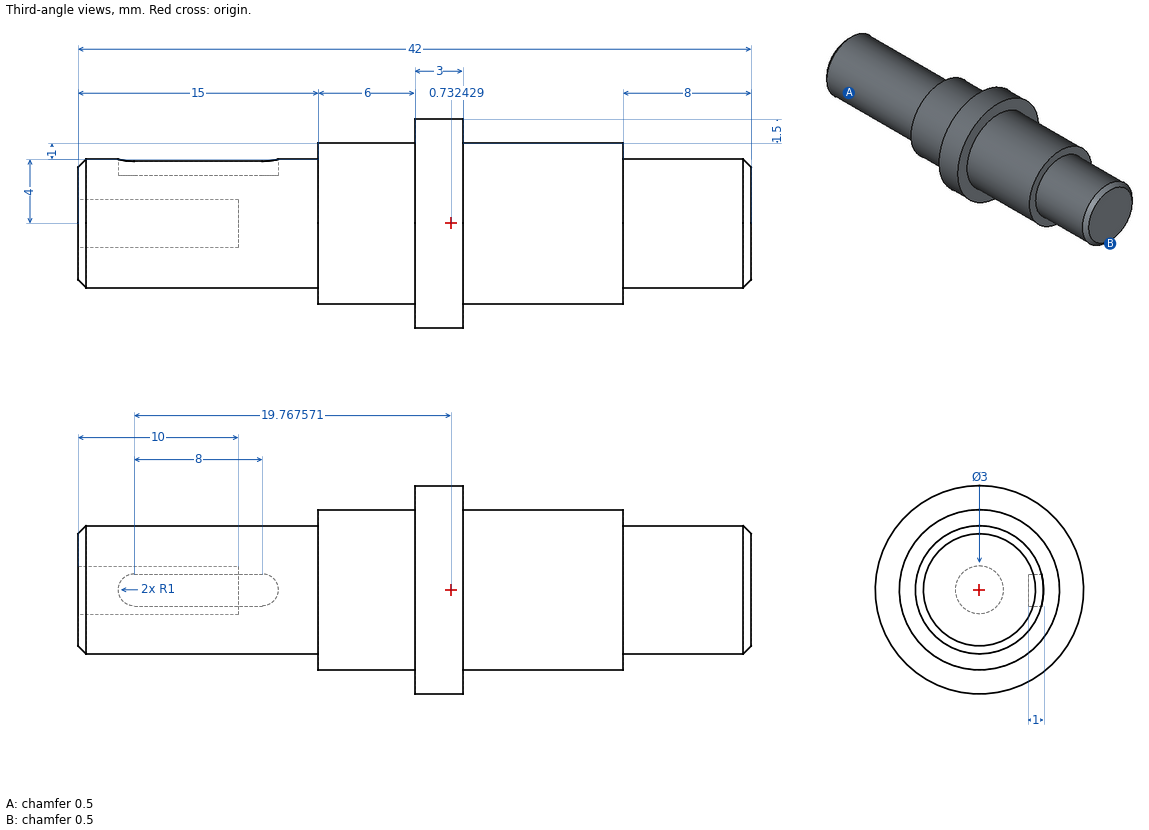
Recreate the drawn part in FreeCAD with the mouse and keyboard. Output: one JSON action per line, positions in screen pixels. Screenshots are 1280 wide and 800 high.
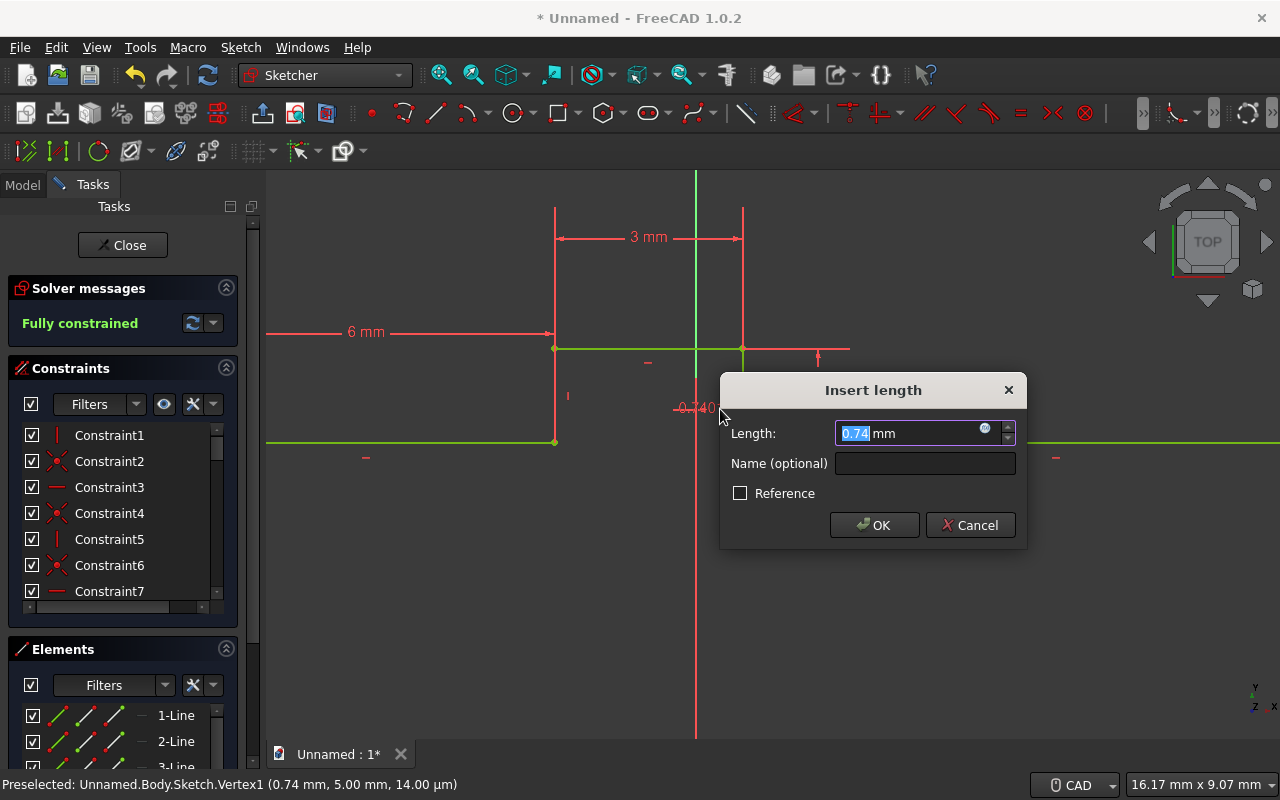
{"action": "type", "text": "0.732429"}
{"action": "key", "text": "Return"}
{"action": "key", "text": "Escape"}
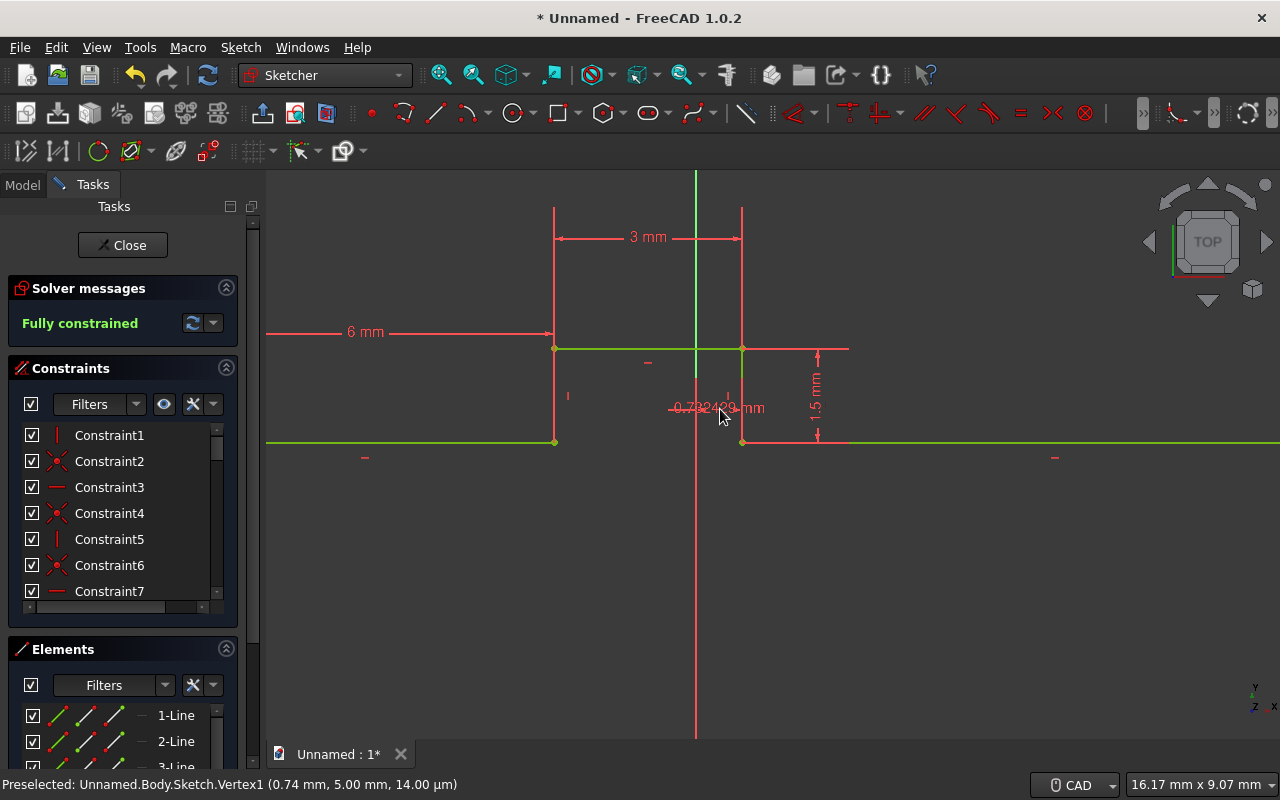
{"action": "left_click", "coordinate": [123, 245]}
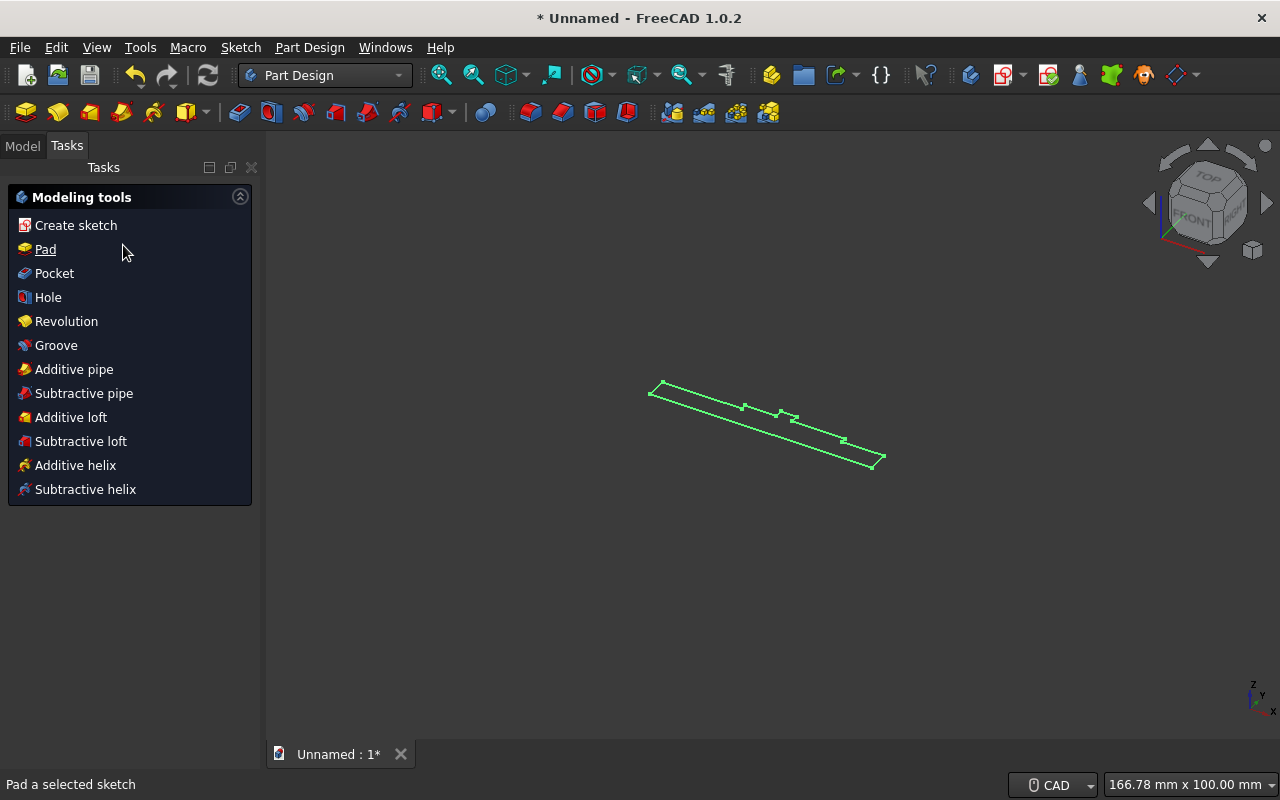
{"action": "left_click", "coordinate": [58, 112]}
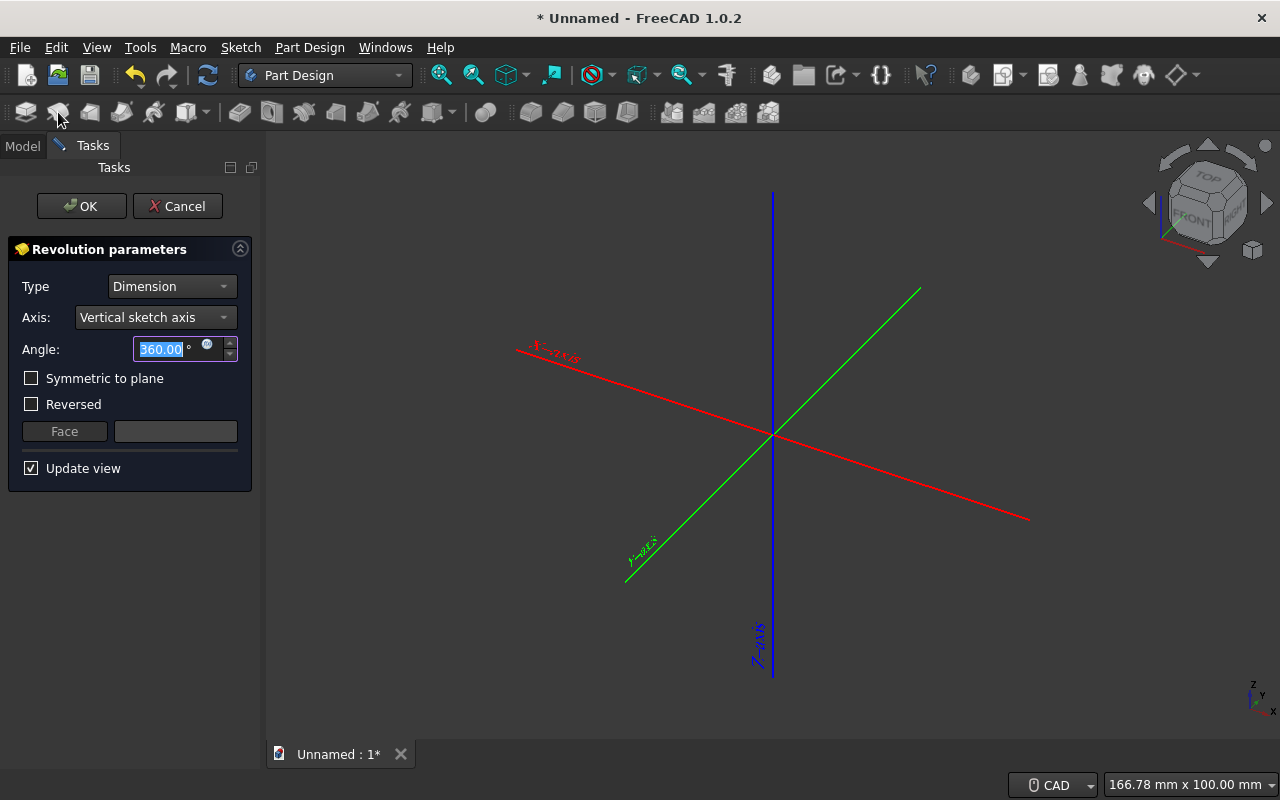
{"action": "left_click", "coordinate": [156, 318]}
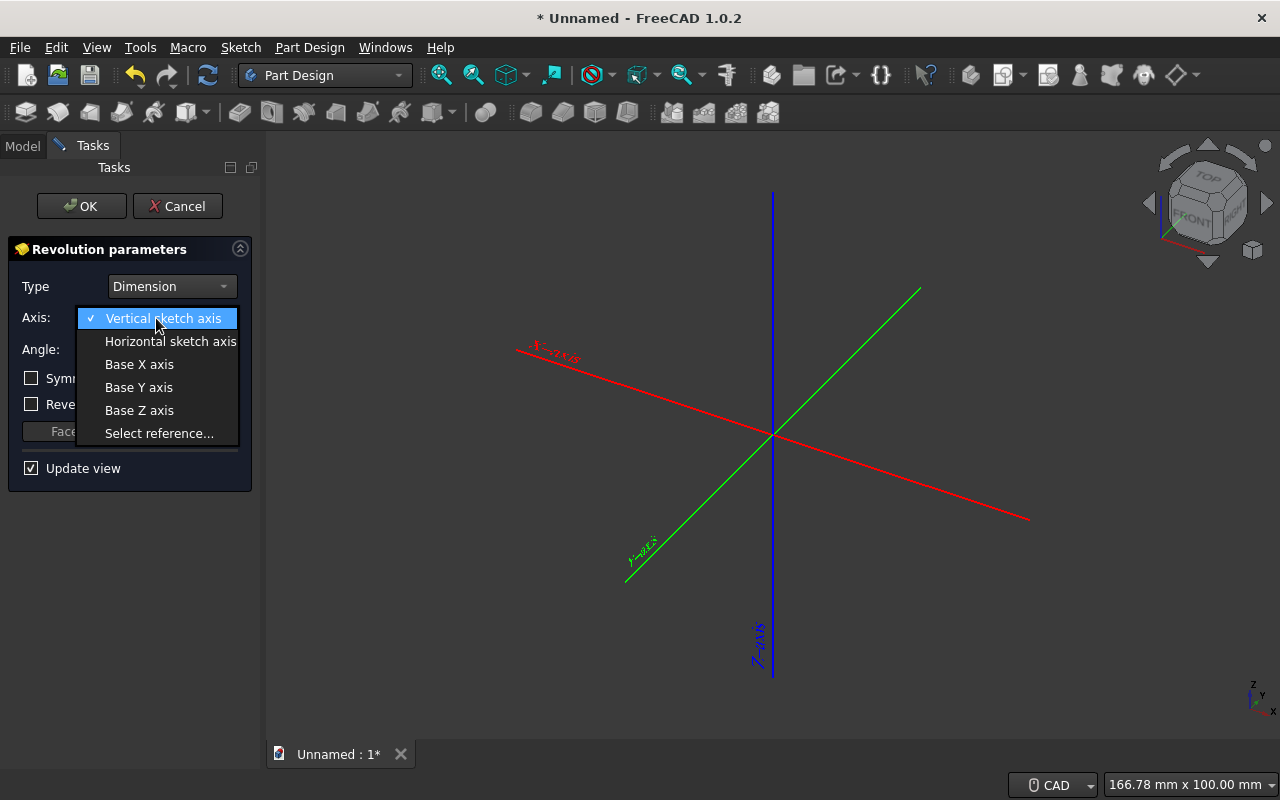
{"action": "left_click", "coordinate": [156, 342]}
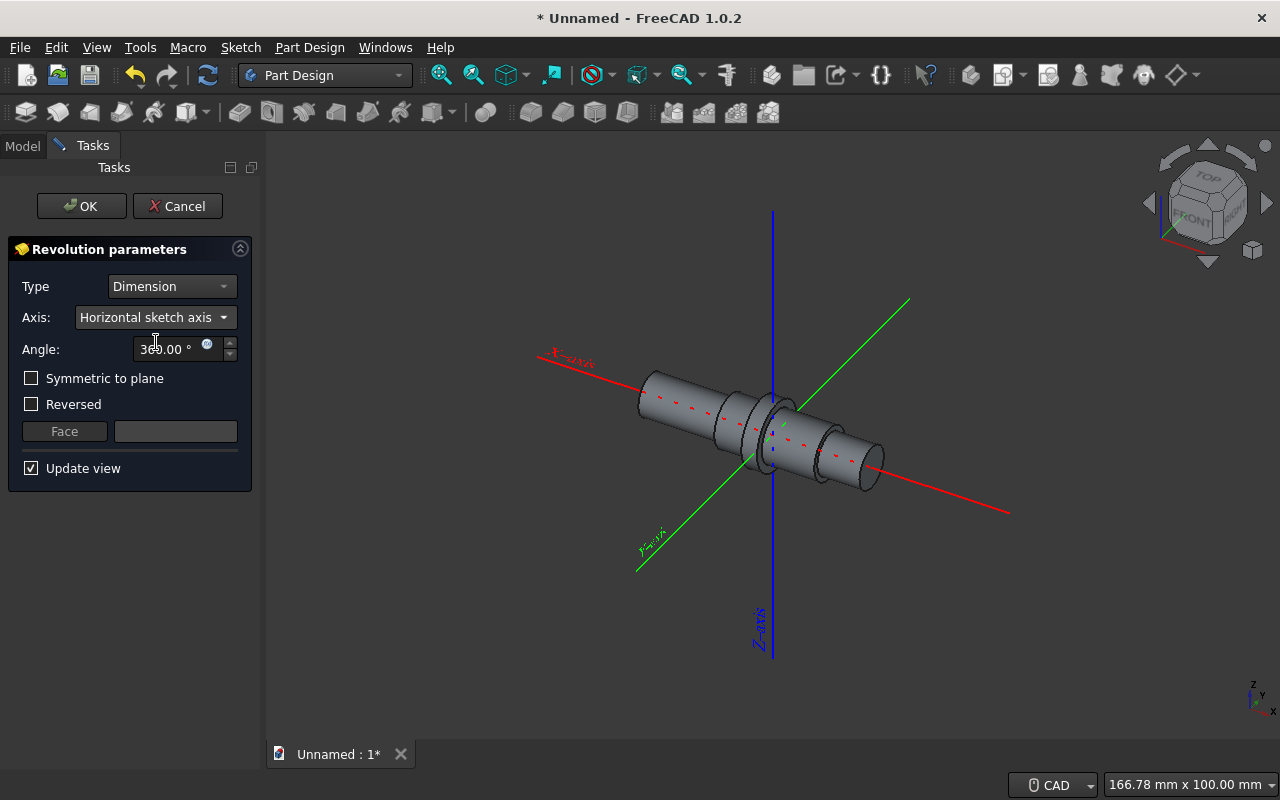
{"action": "left_click", "coordinate": [82, 206]}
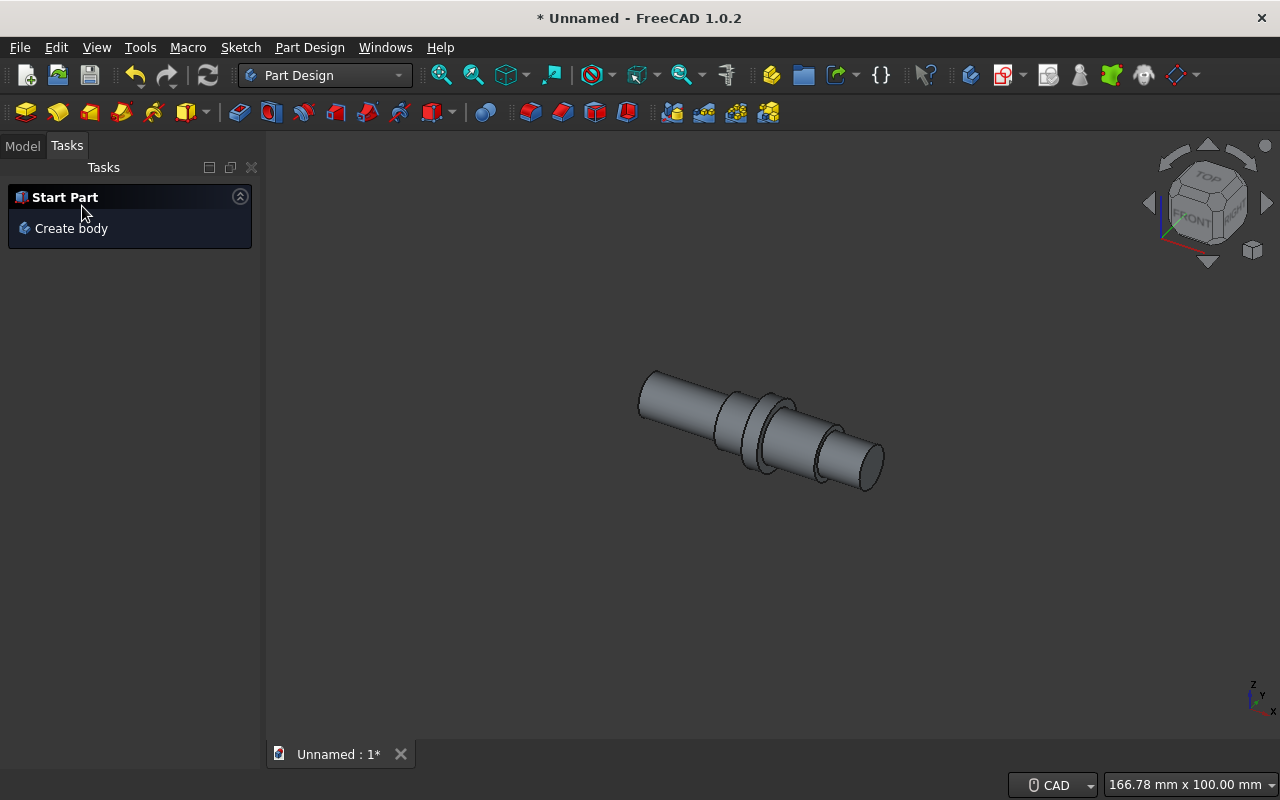
{"action": "left_click", "coordinate": [442, 76]}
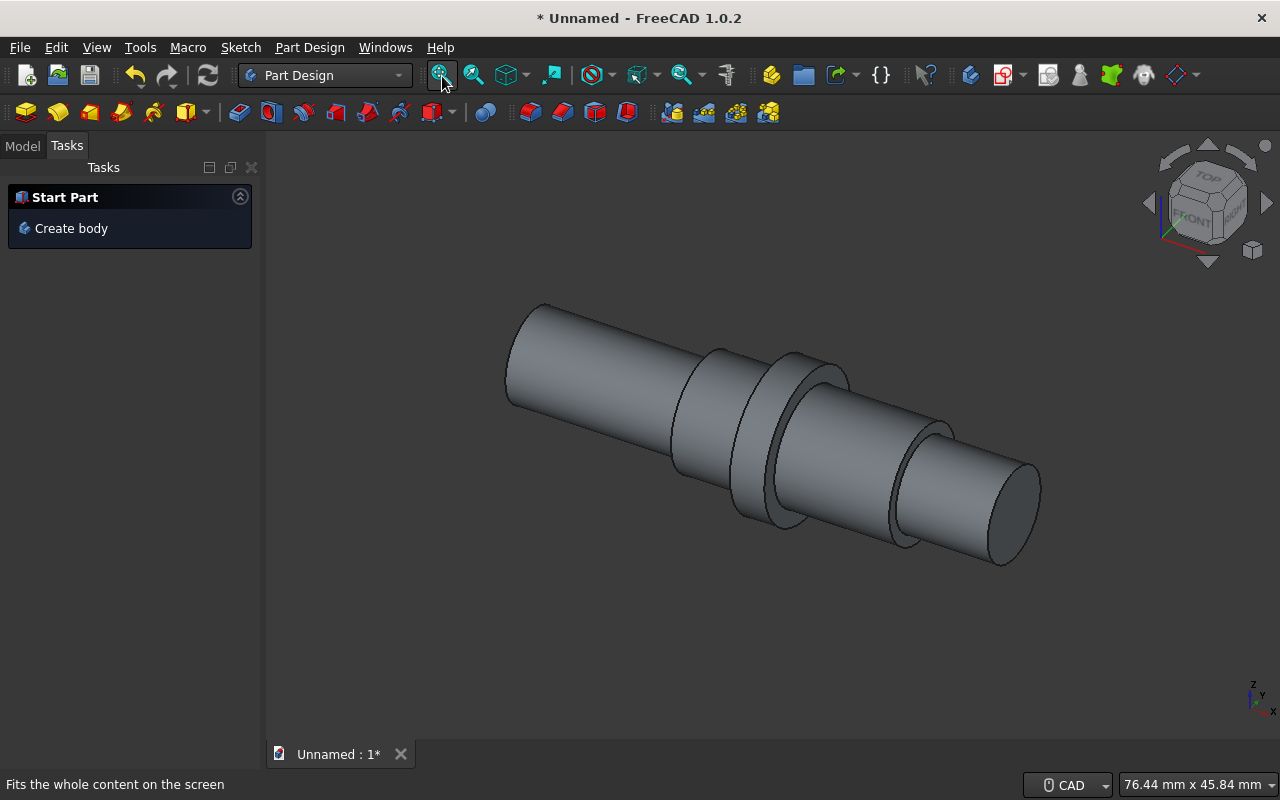
{"action": "left_click", "coordinate": [23, 145]}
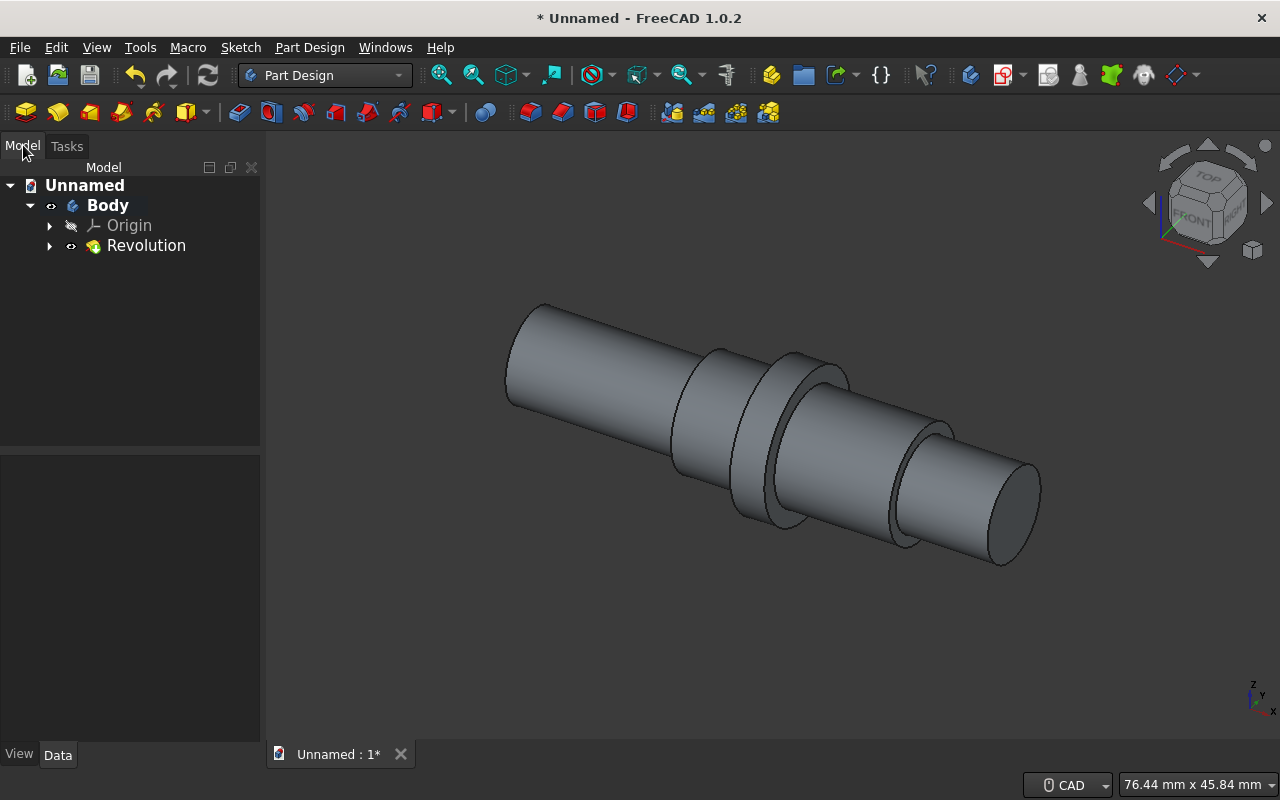
{"action": "left_click", "coordinate": [50, 226]}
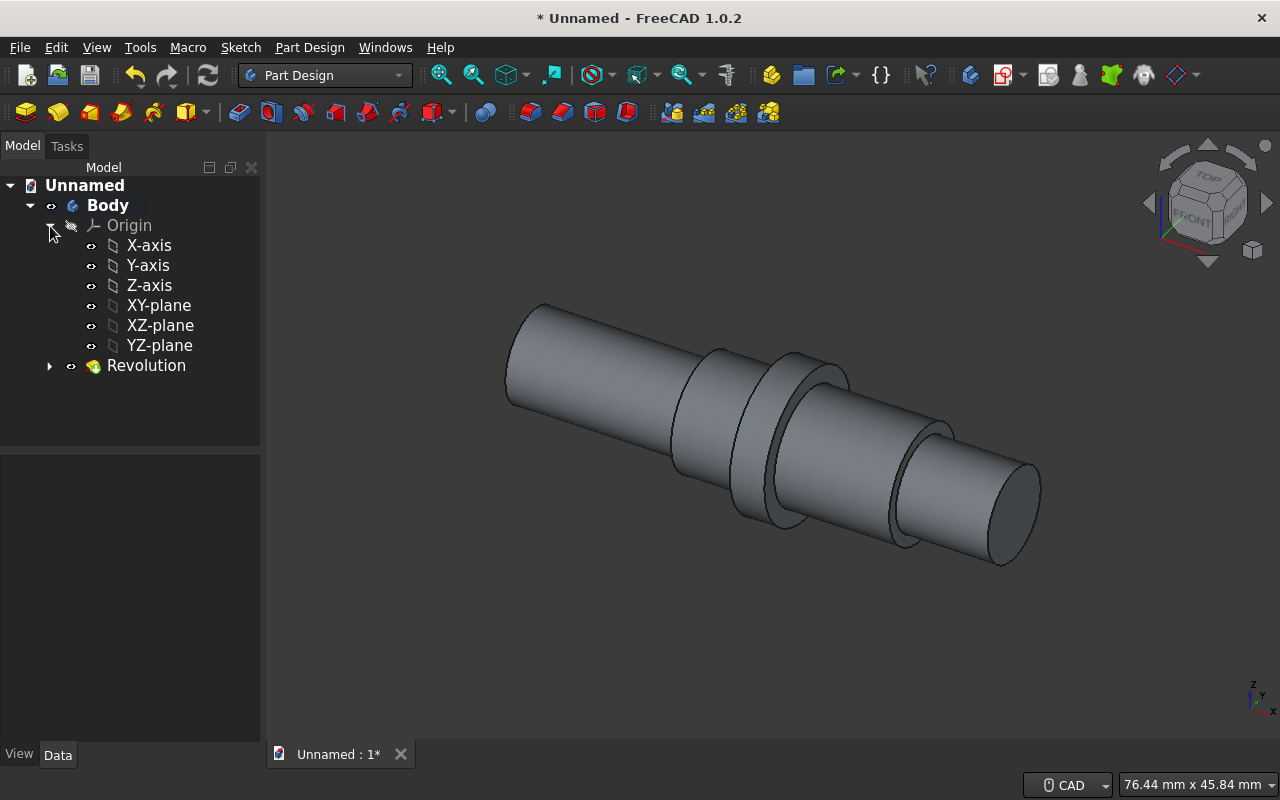
{"action": "left_click", "coordinate": [136, 326]}